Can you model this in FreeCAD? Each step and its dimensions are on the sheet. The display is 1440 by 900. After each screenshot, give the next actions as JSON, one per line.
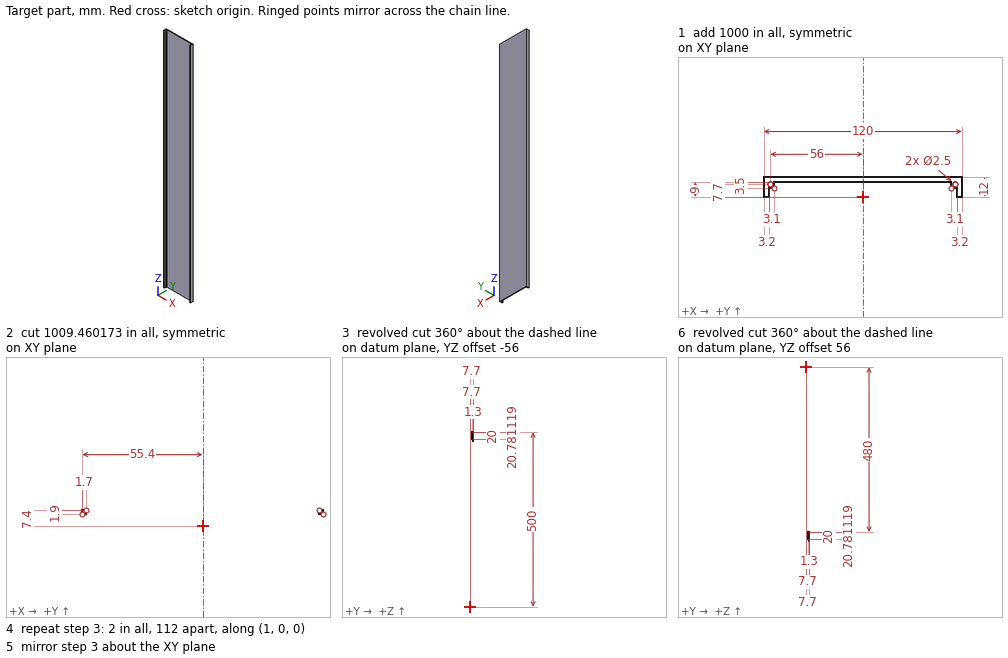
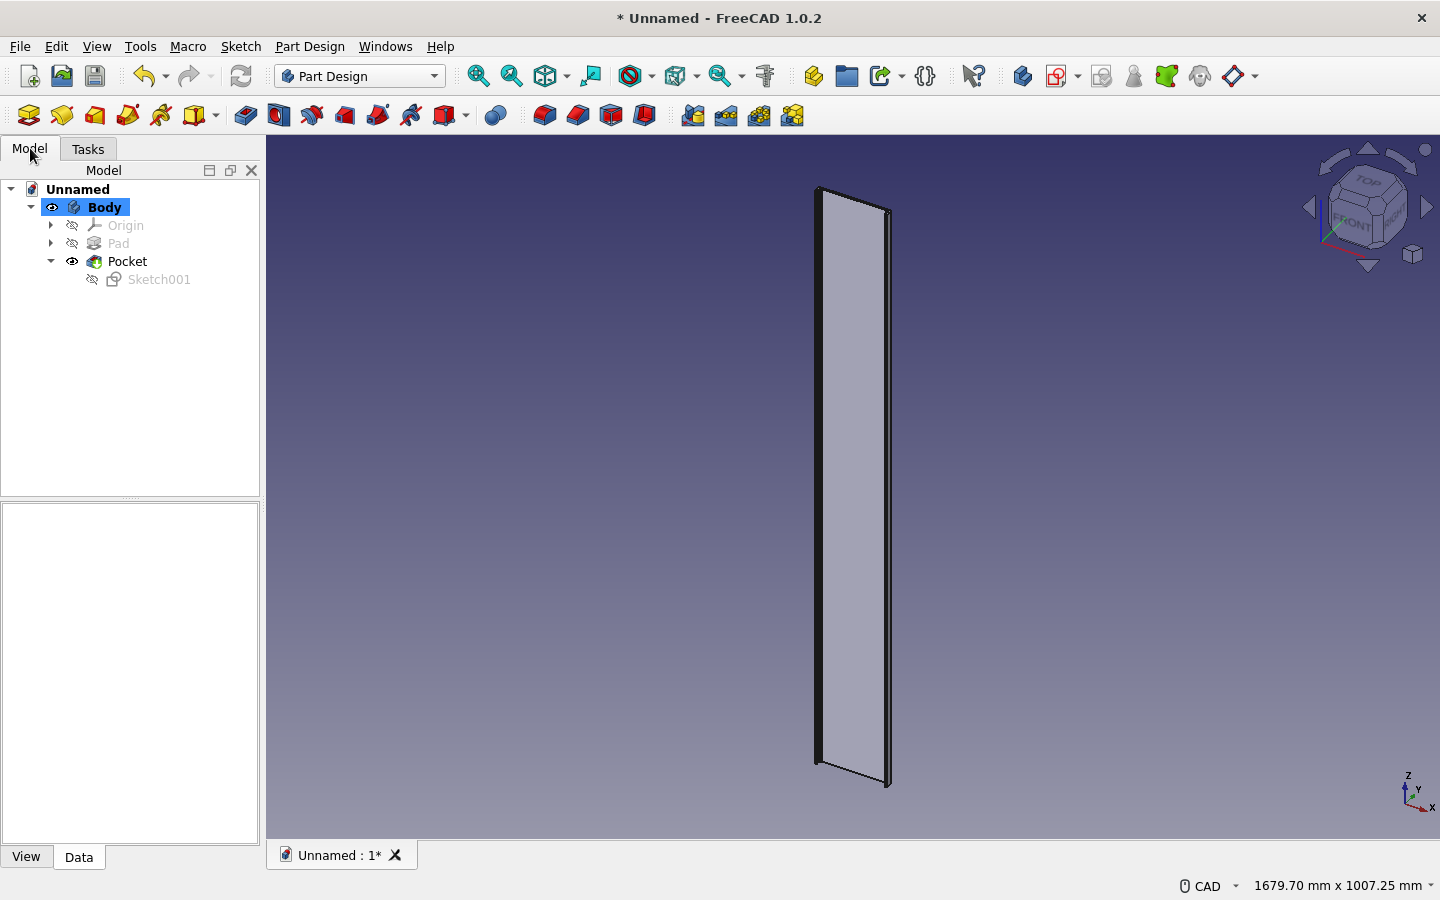
{"action": "left_click", "coordinate": [51, 225]}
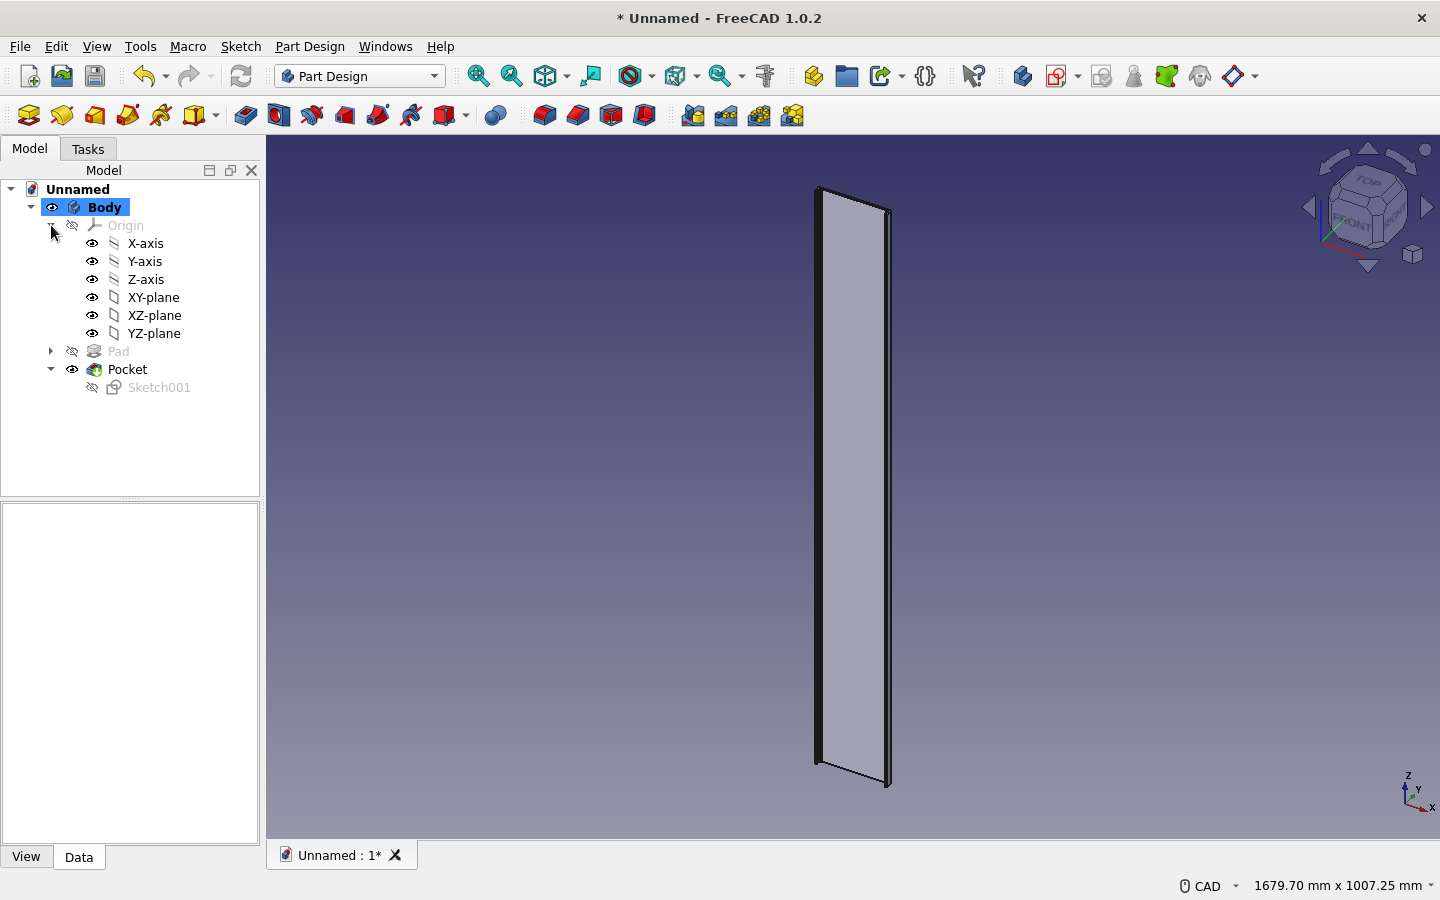
{"action": "left_click", "coordinate": [137, 333]}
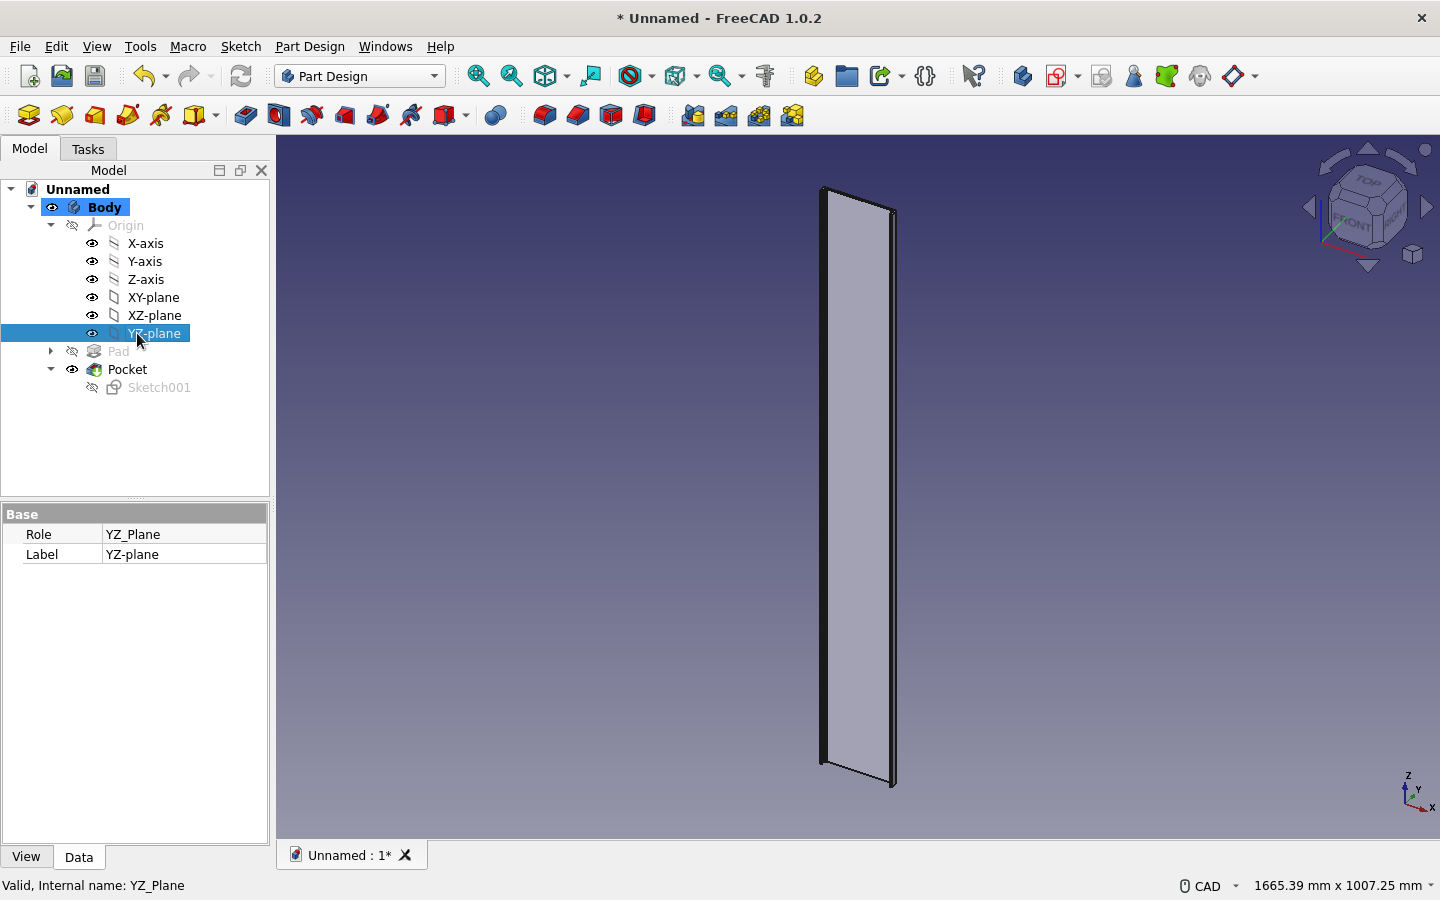
{"action": "left_click", "coordinate": [1232, 76]}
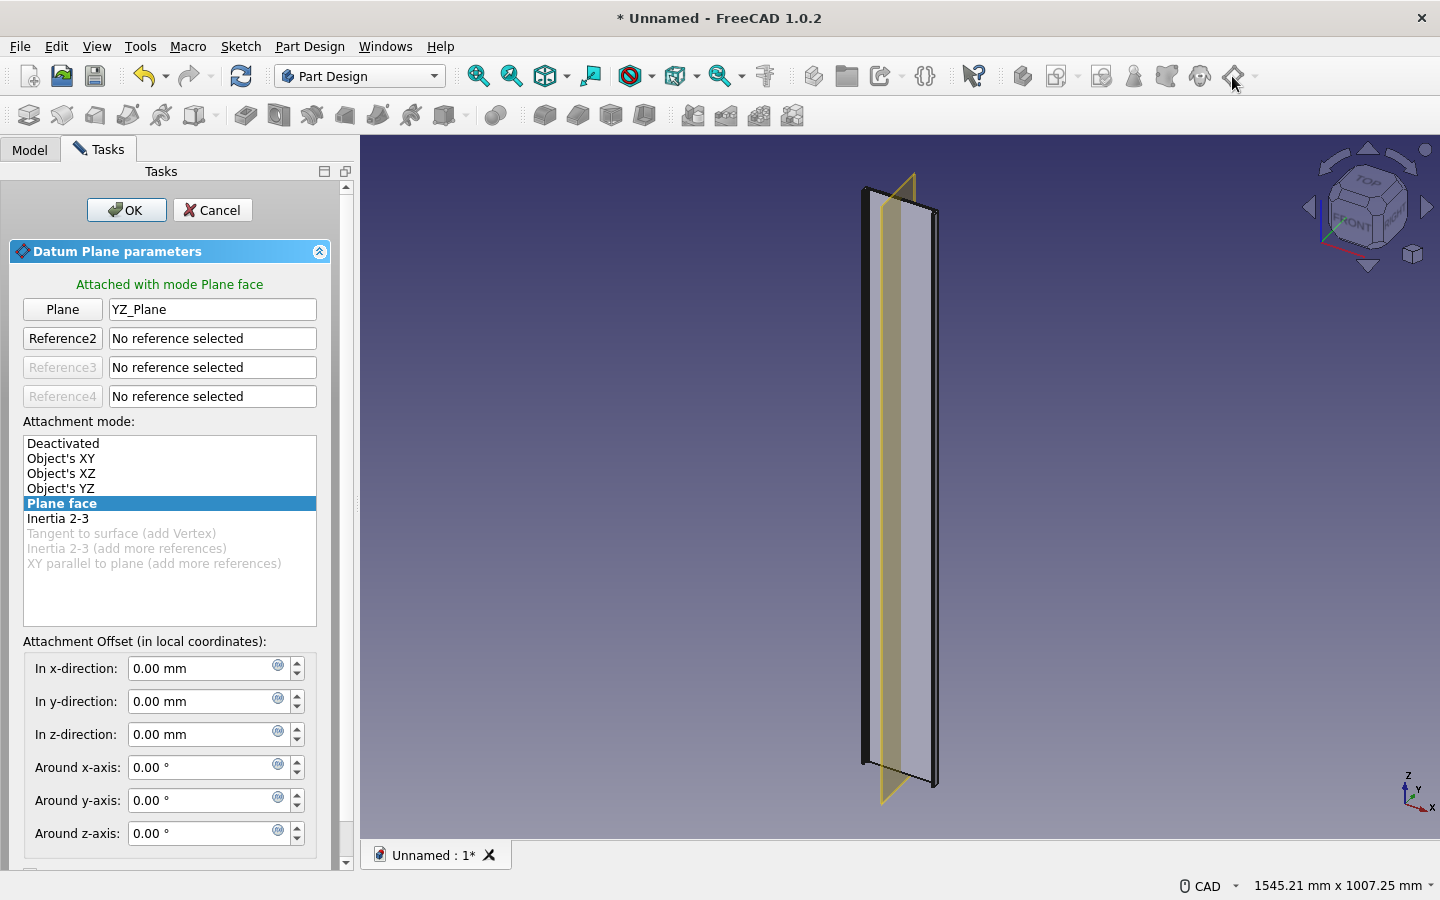
{"action": "triple_click", "coordinate": [210, 734]}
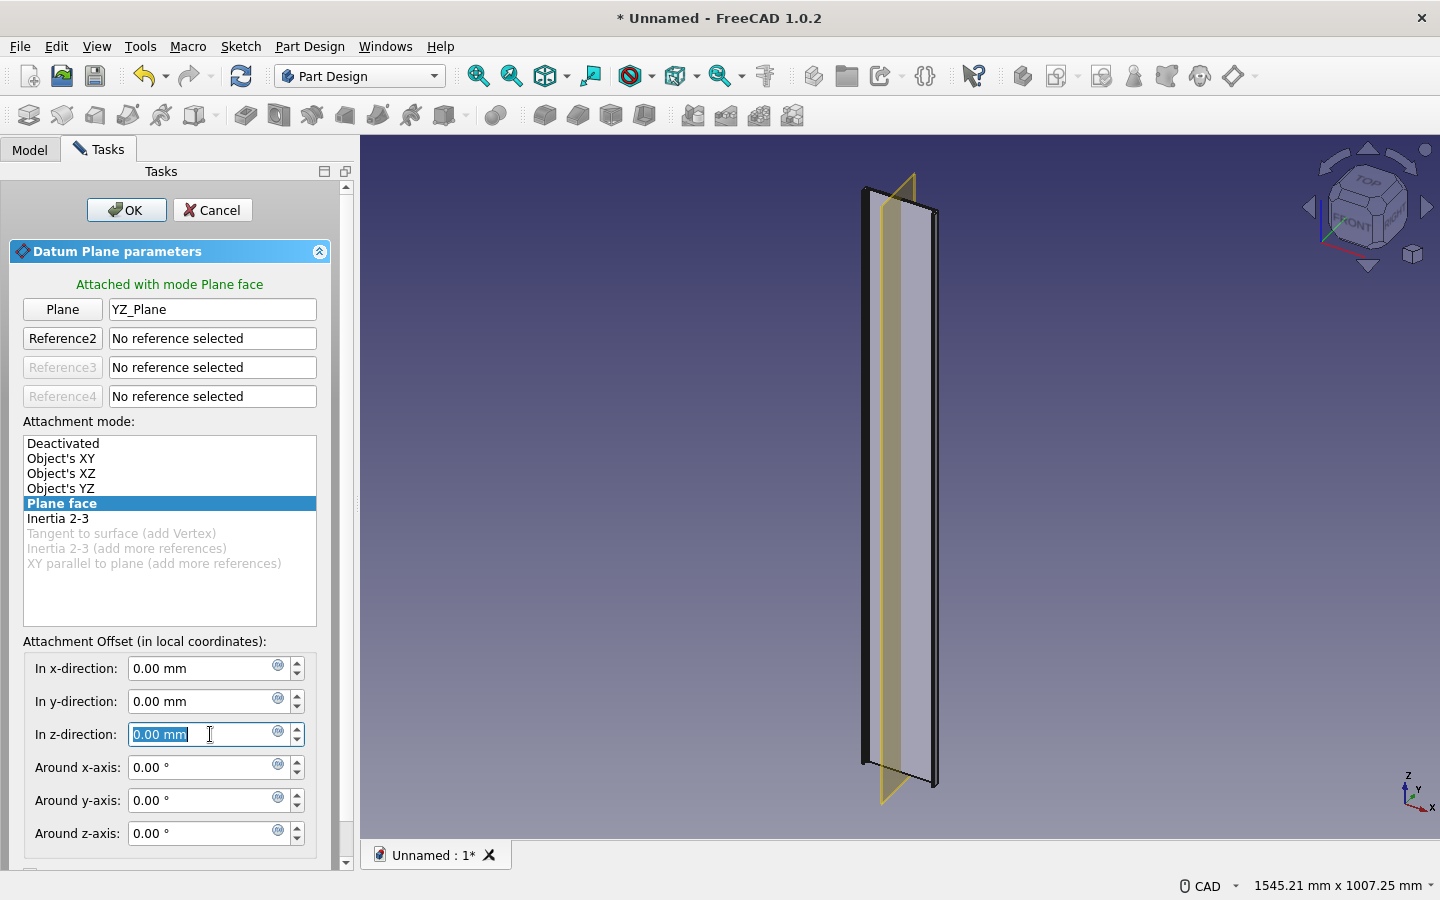
{"action": "type", "text": "-56"}
{"action": "key", "text": "Tab"}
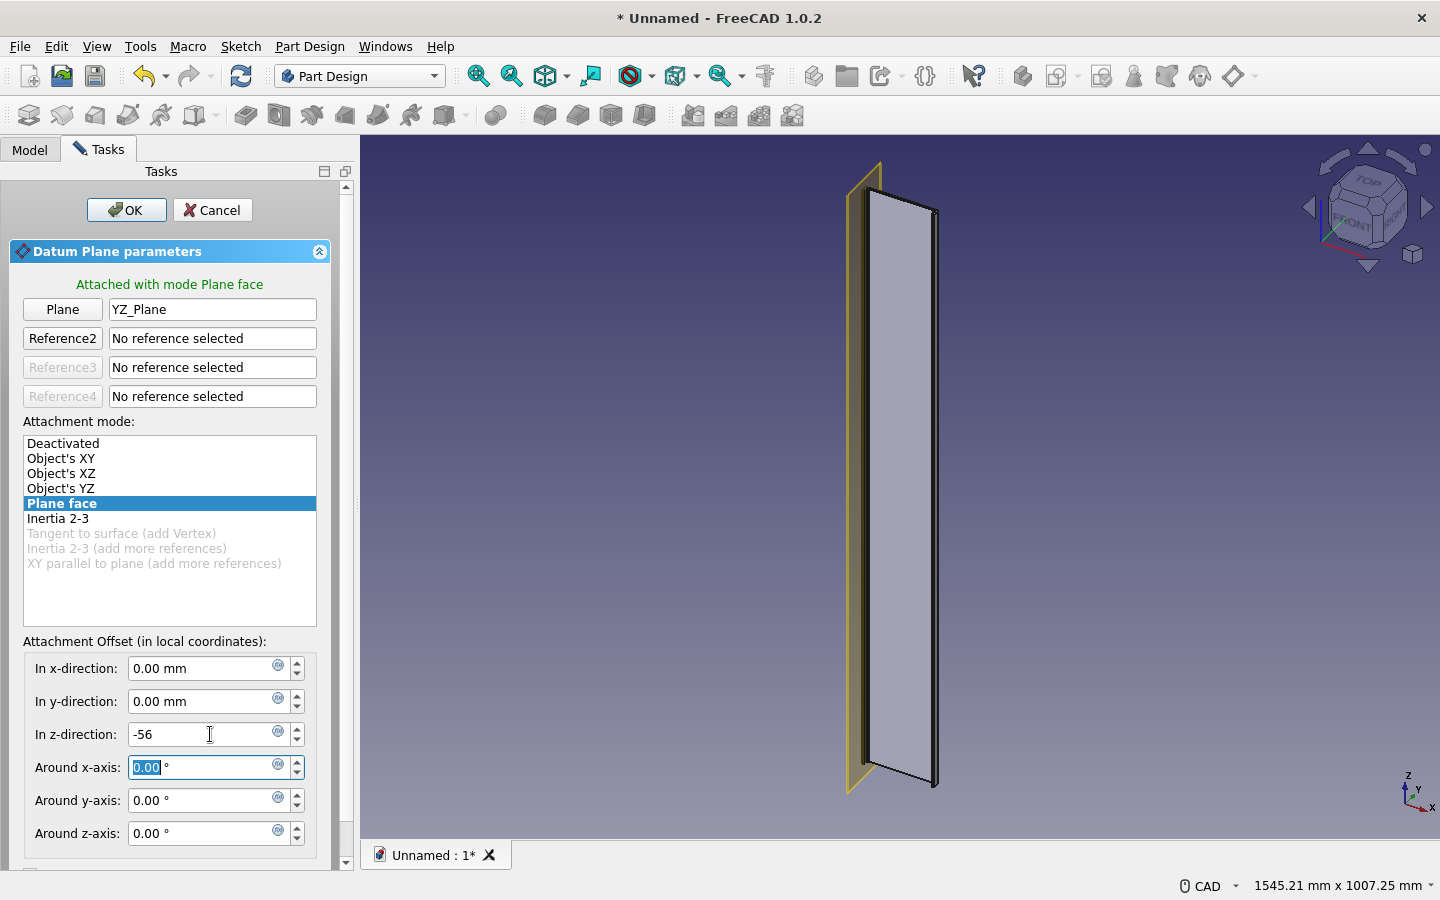
{"action": "left_click", "coordinate": [127, 210]}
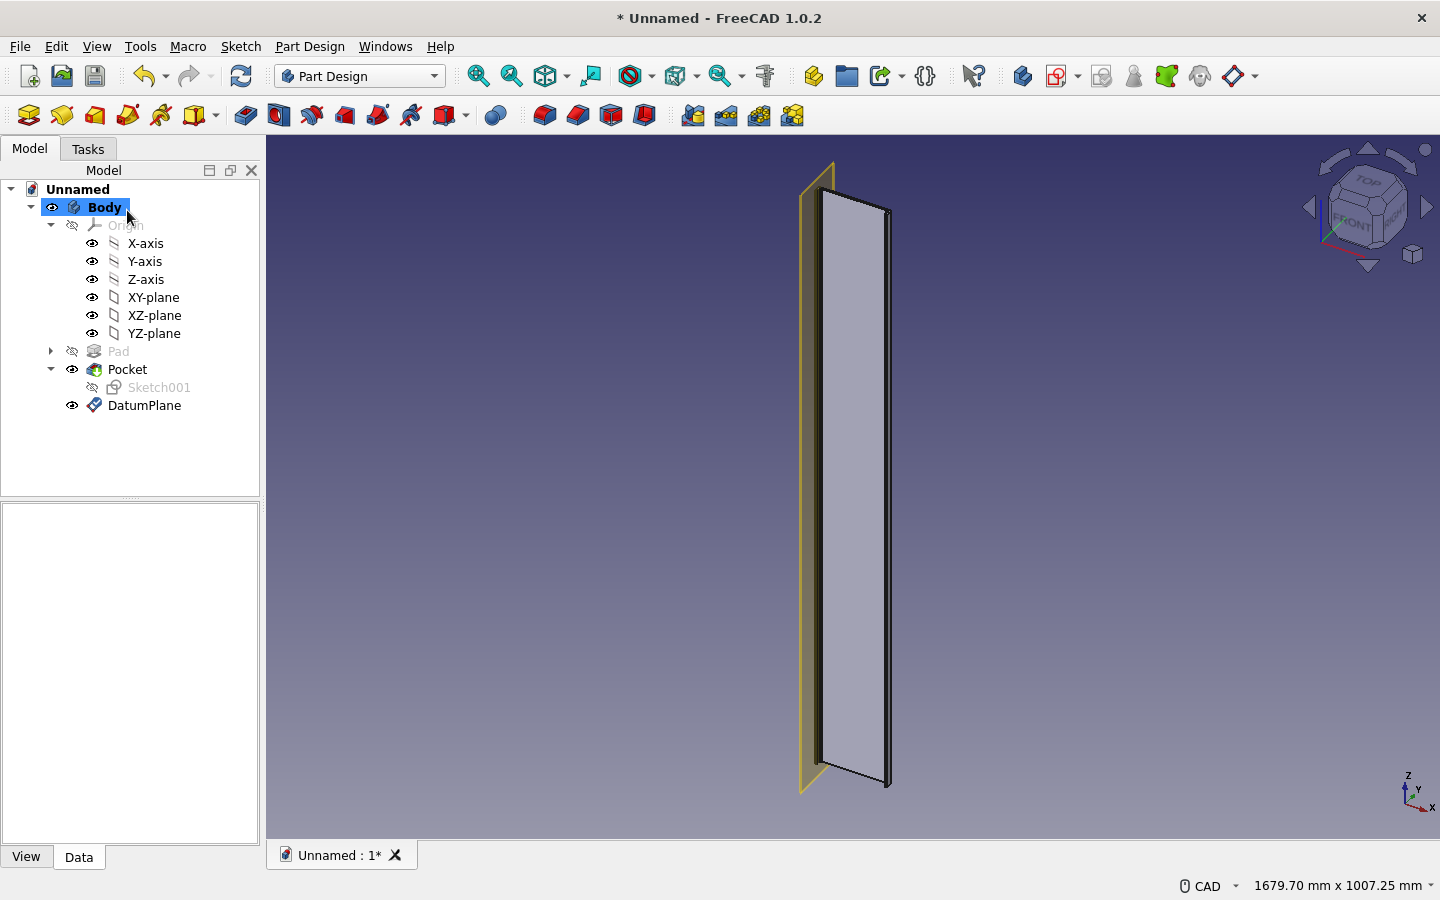
{"action": "left_click", "coordinate": [117, 405]}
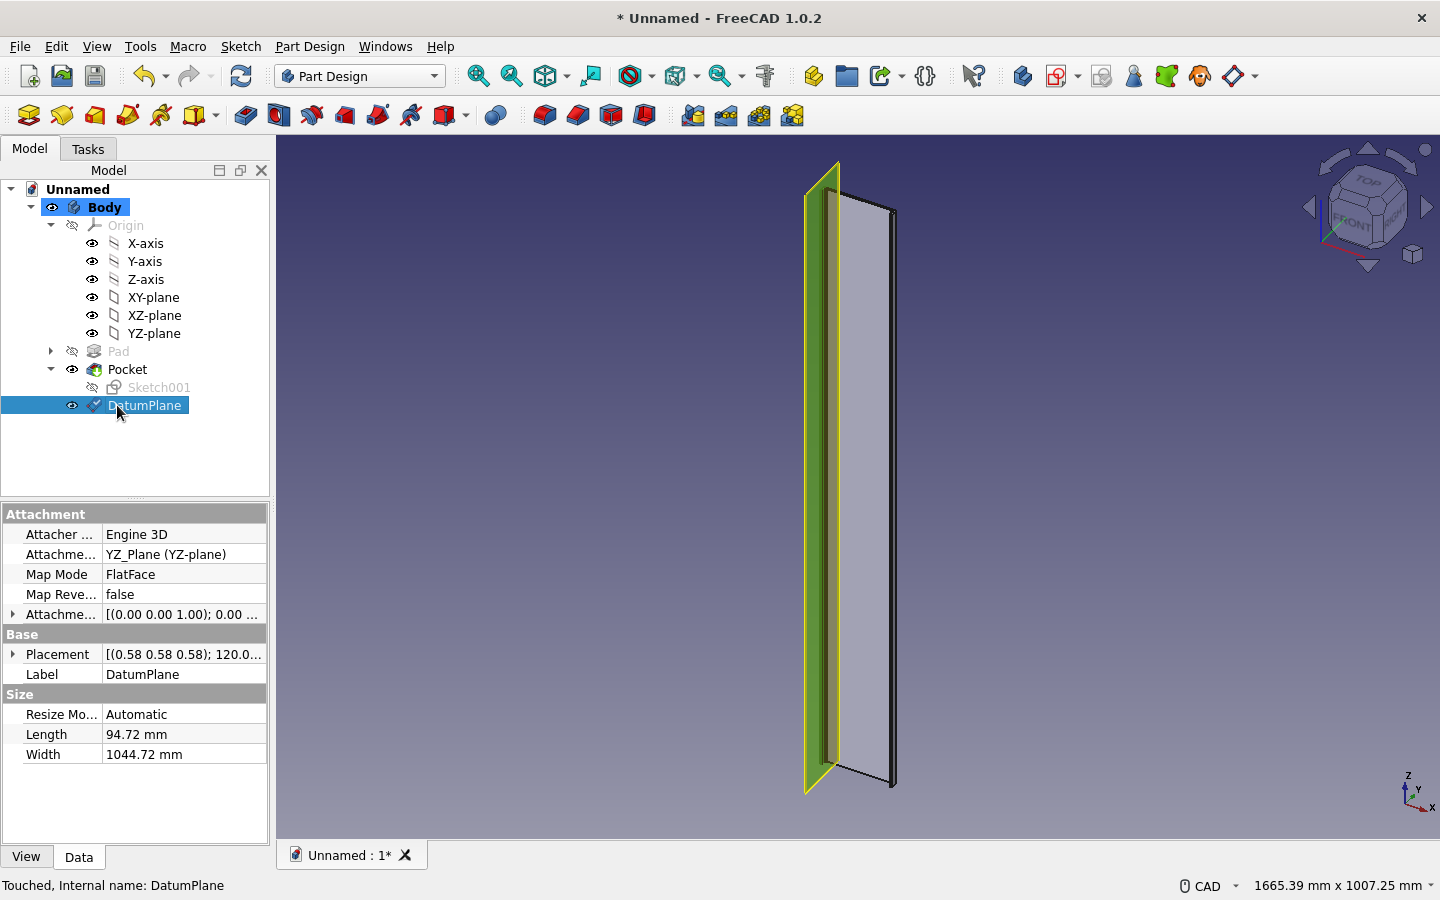
{"action": "left_click", "coordinate": [1056, 76]}